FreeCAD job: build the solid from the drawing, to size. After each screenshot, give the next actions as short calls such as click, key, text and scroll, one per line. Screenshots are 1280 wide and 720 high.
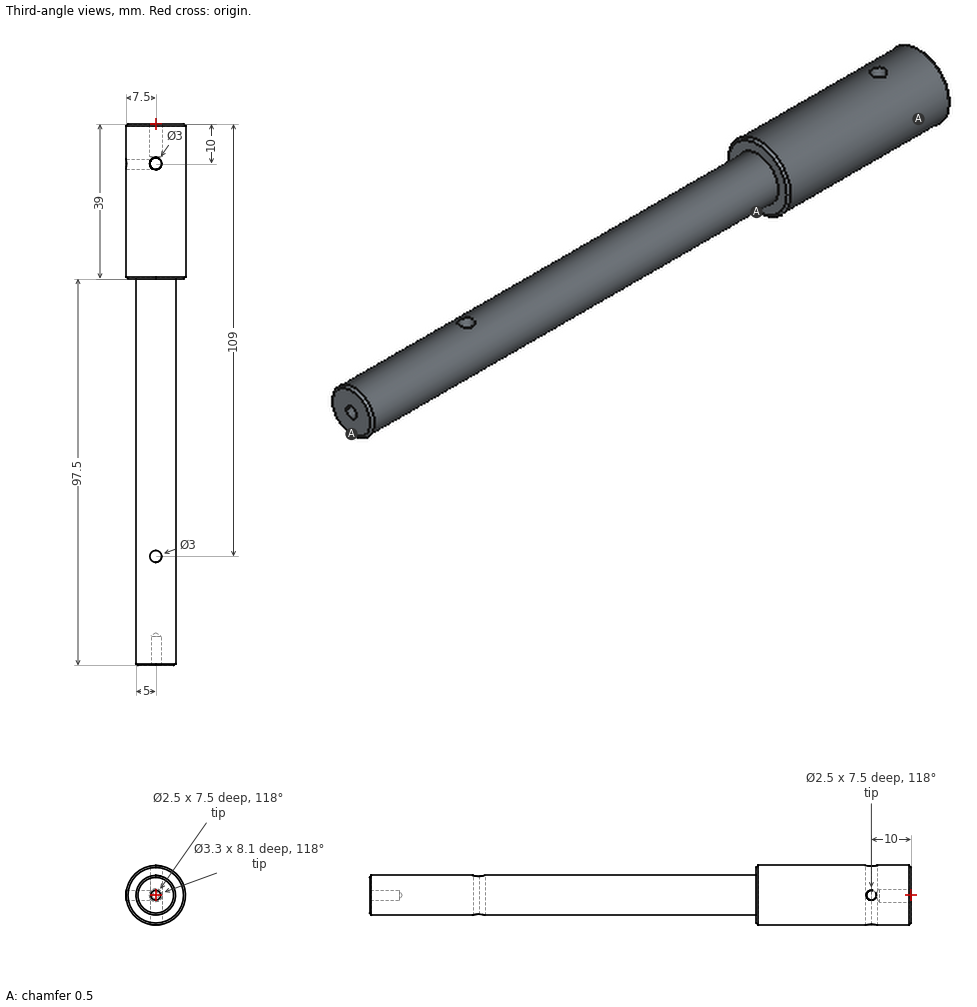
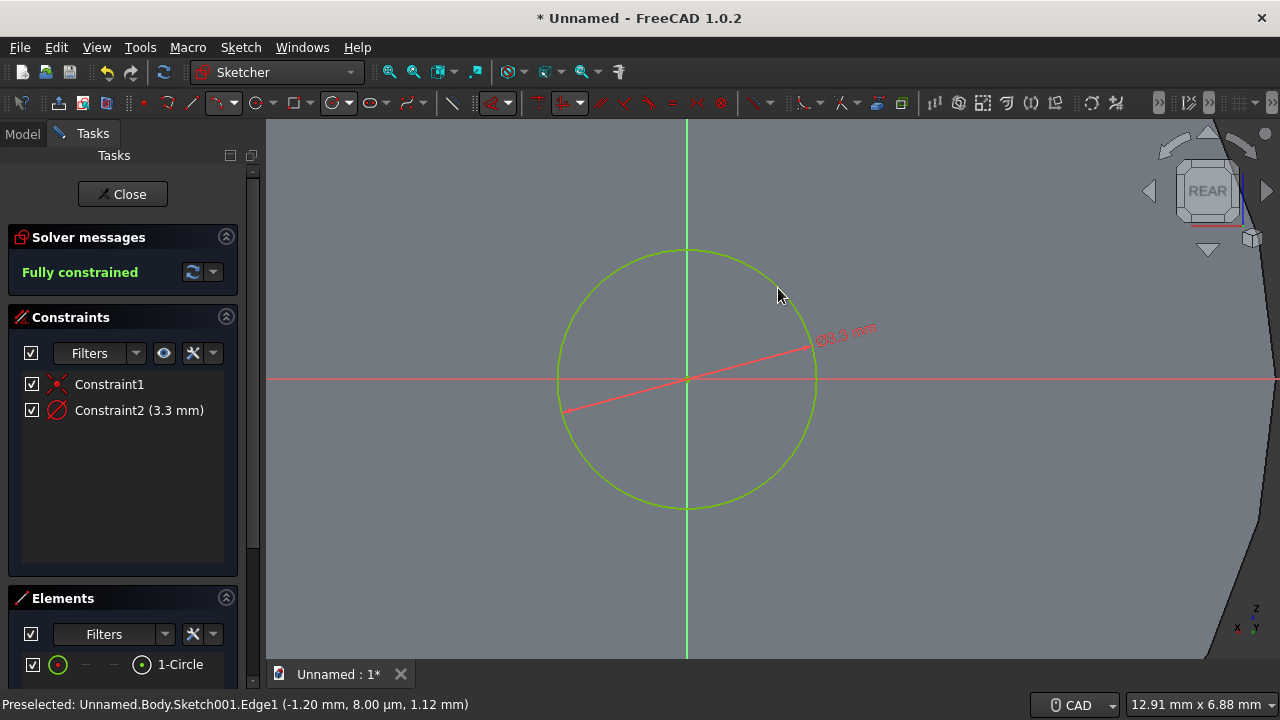
click(123, 194)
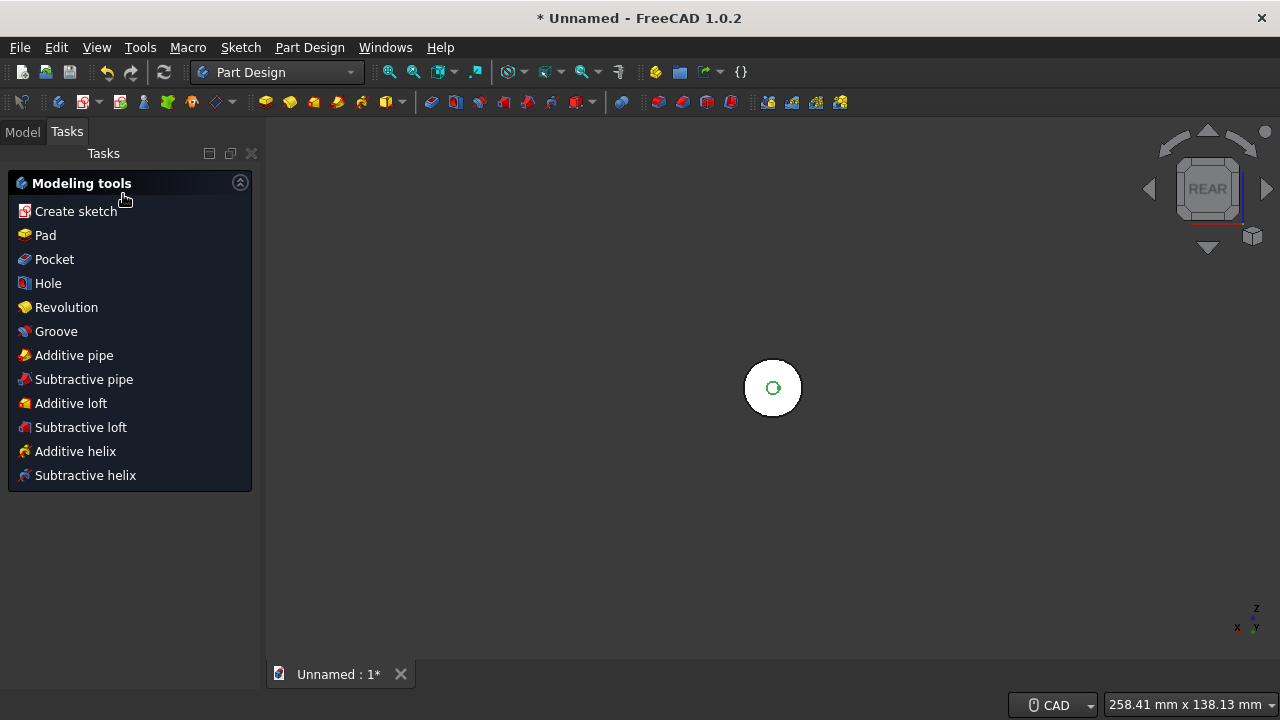
click(456, 102)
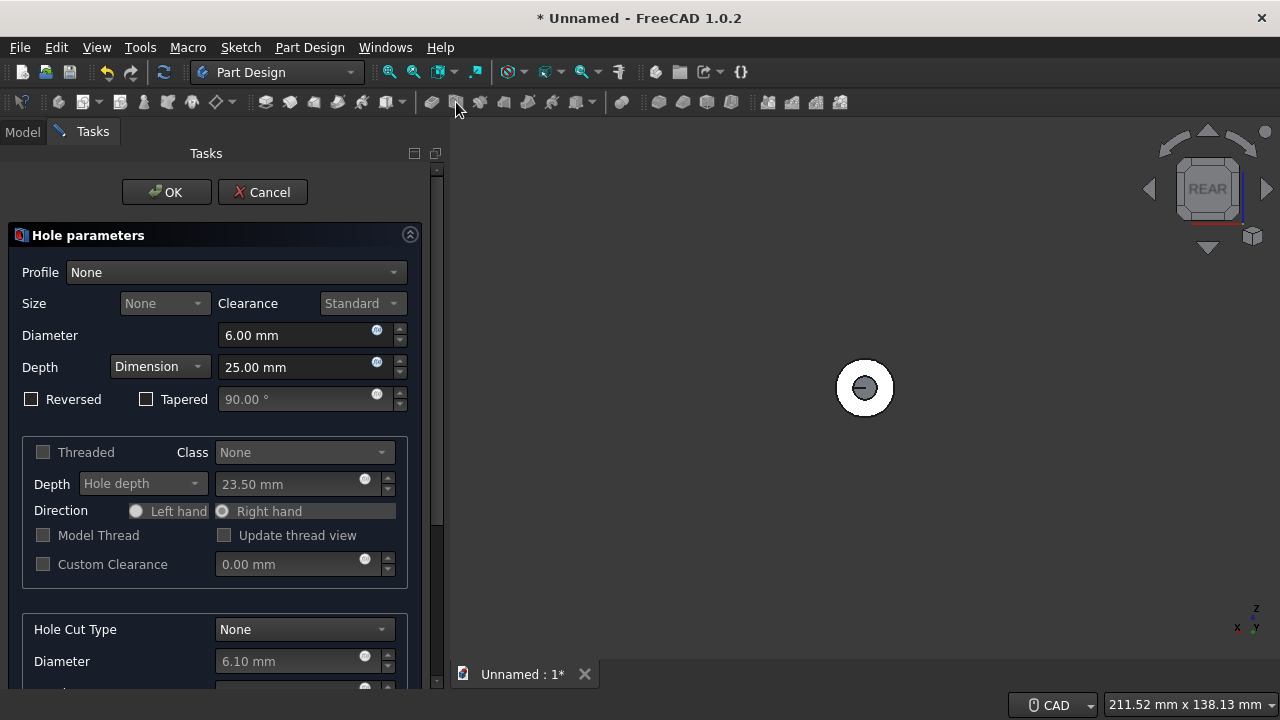
triple_click(305, 335)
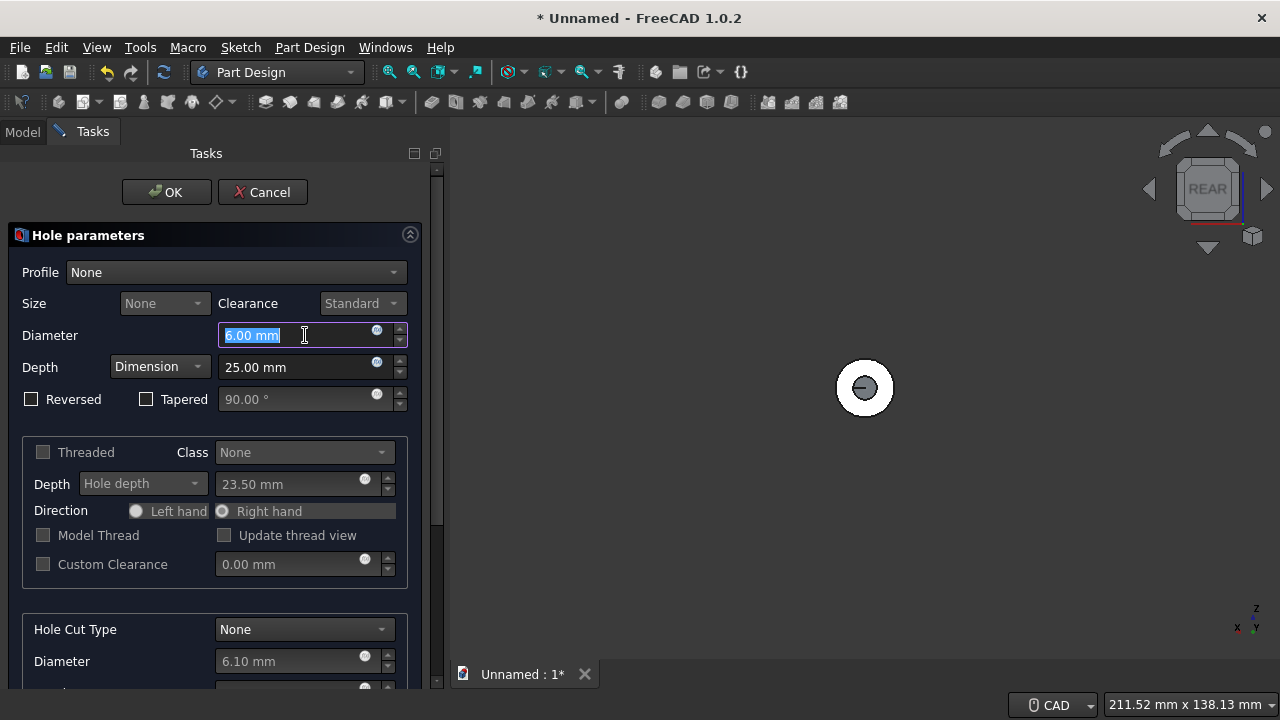
text(3.3)
key(Tab)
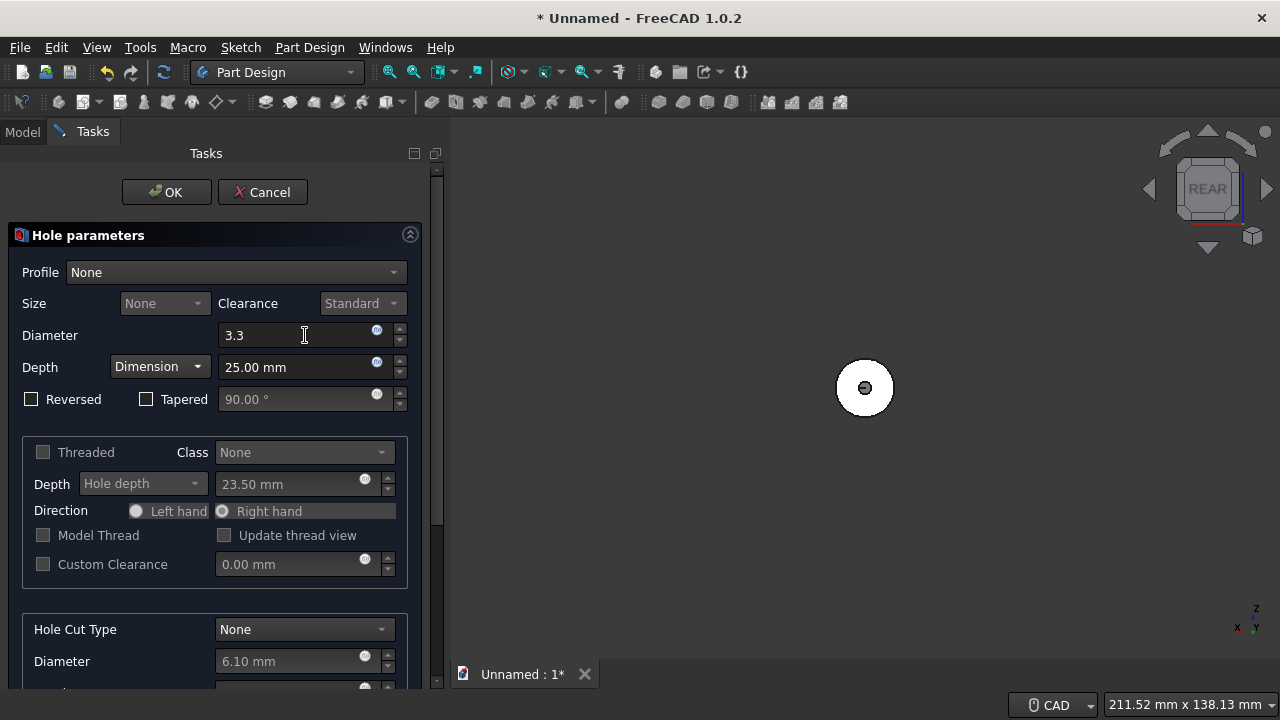
triple_click(305, 367)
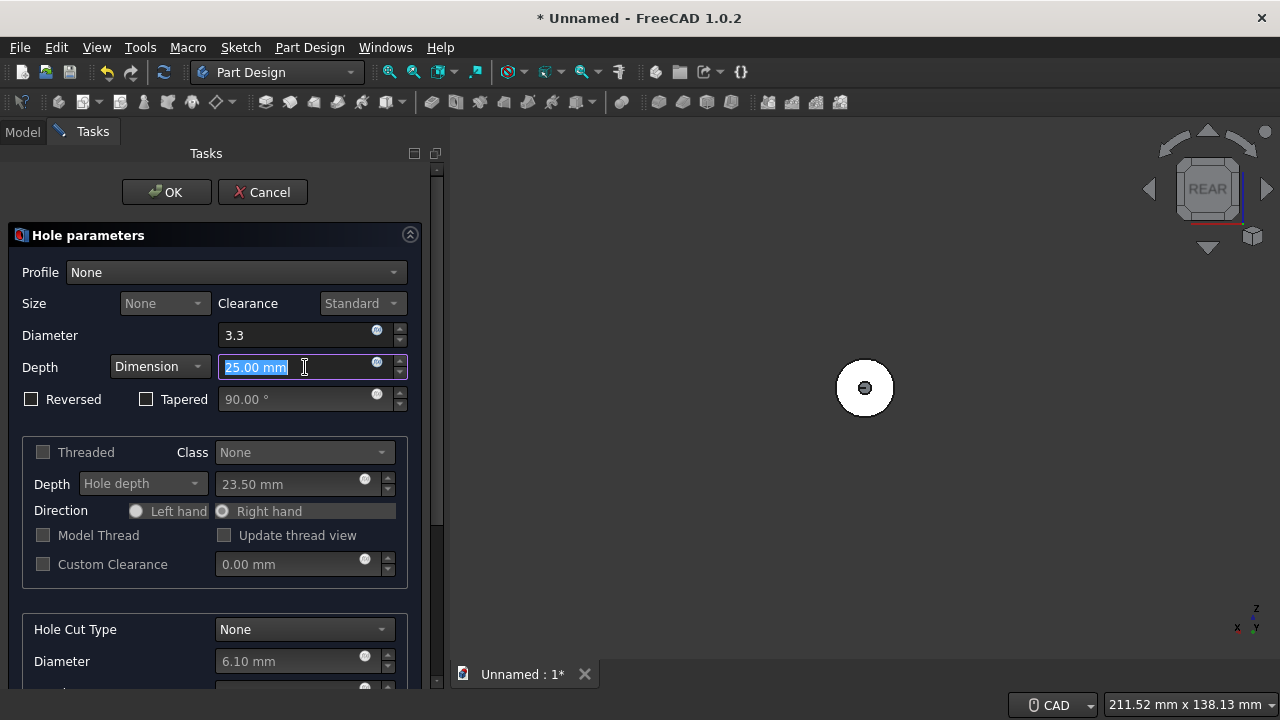
text(8.1)
key(Tab)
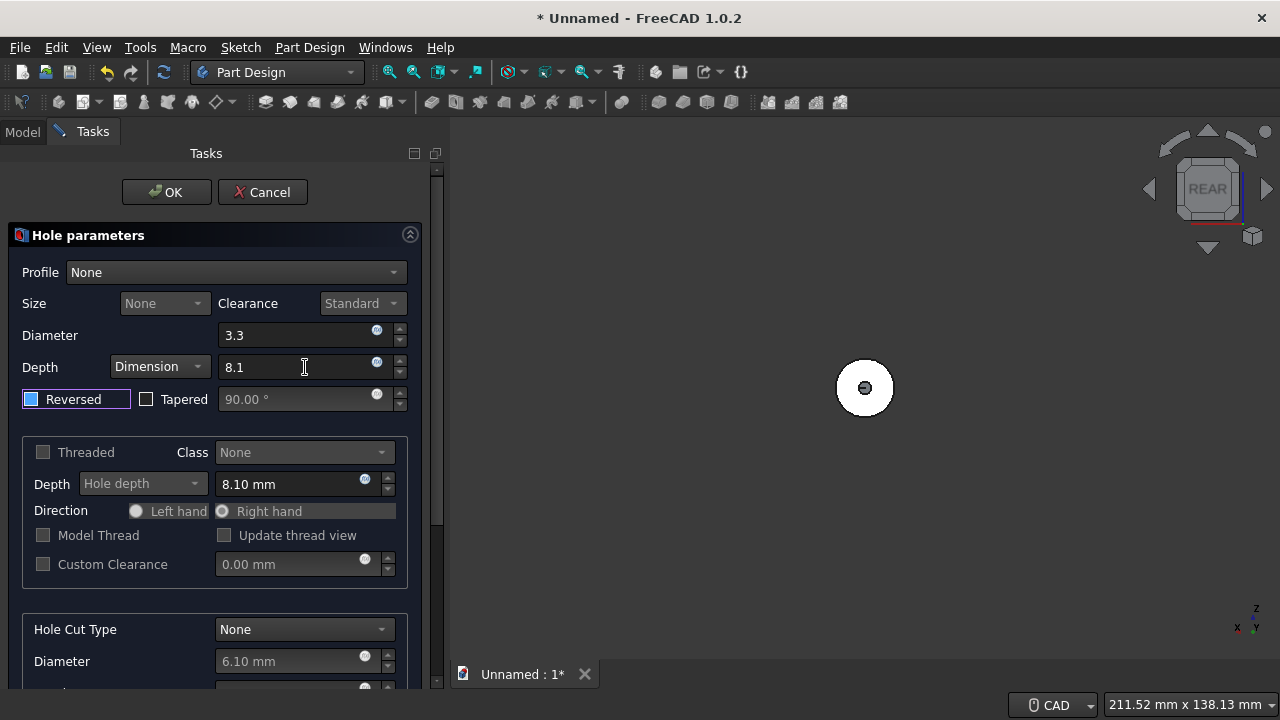
click(167, 192)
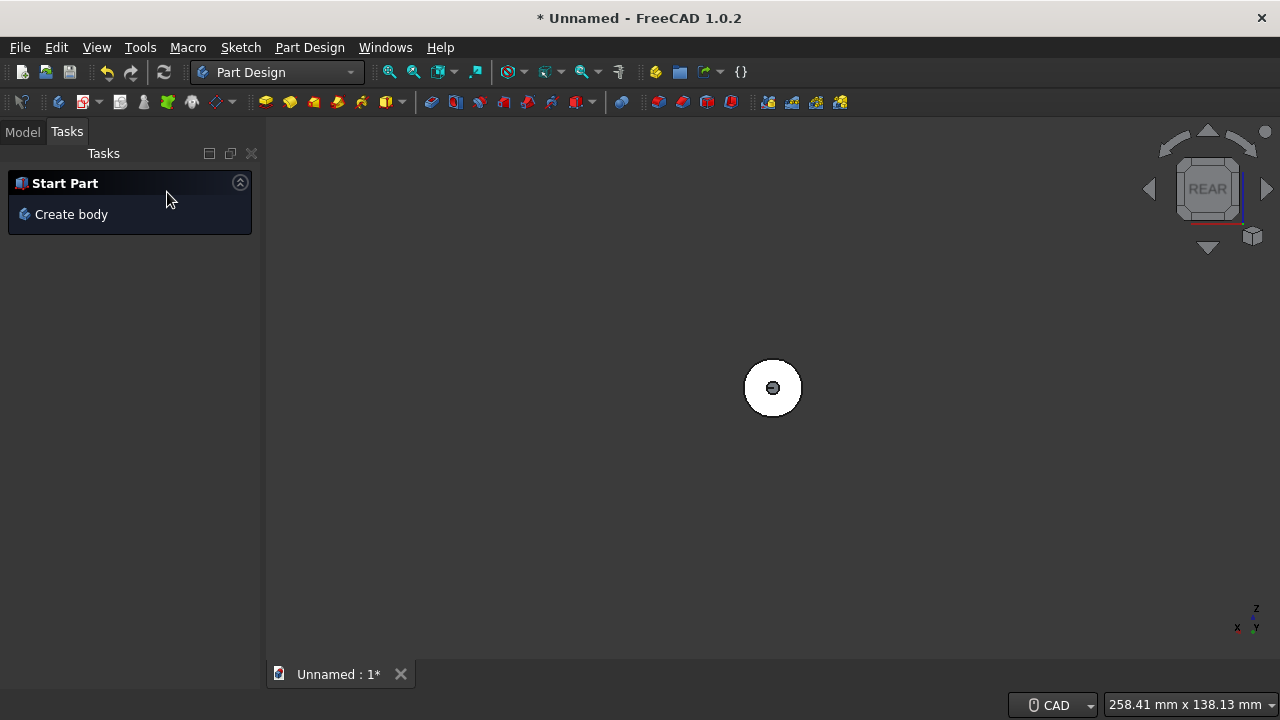
click(390, 72)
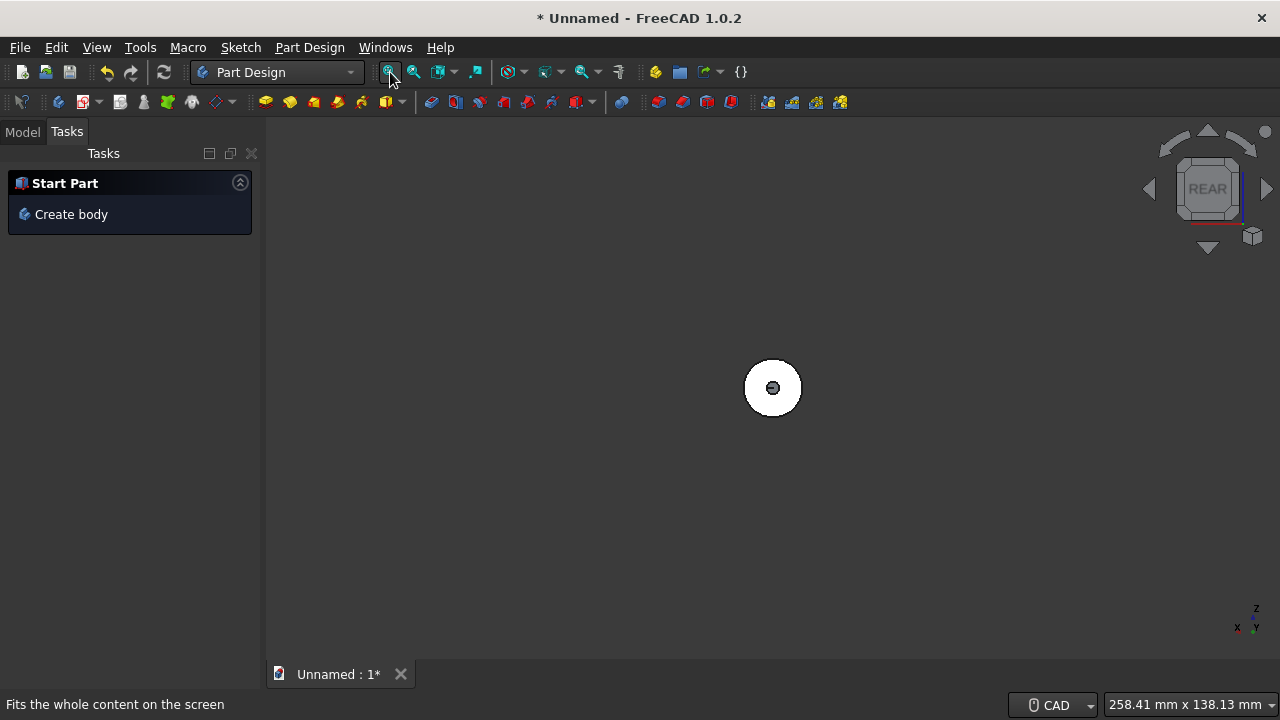
click(84, 102)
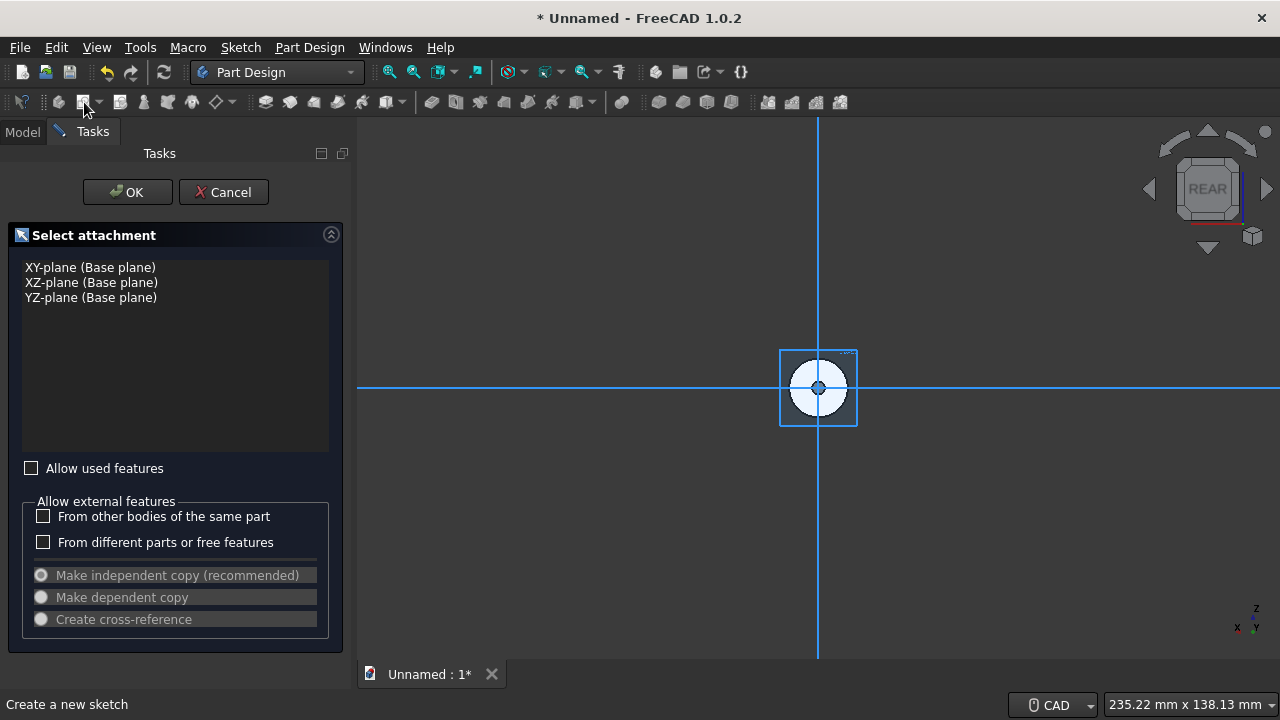
click(82, 268)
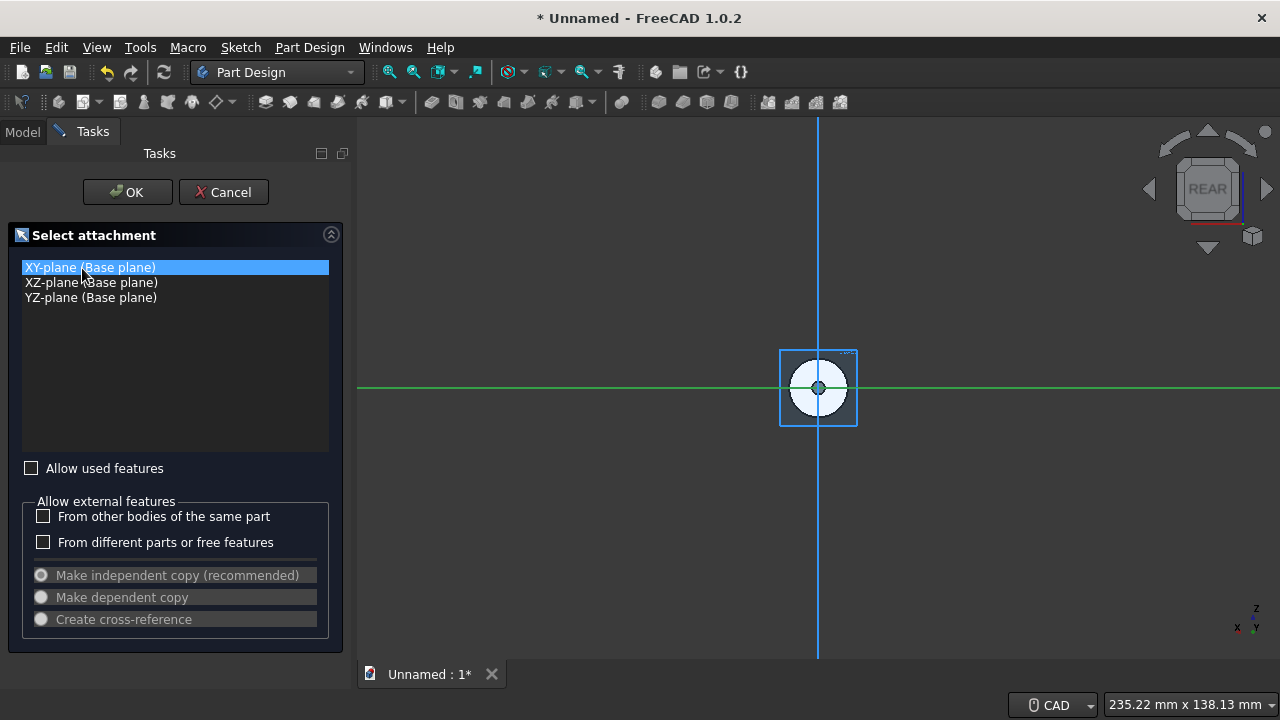
click(128, 192)